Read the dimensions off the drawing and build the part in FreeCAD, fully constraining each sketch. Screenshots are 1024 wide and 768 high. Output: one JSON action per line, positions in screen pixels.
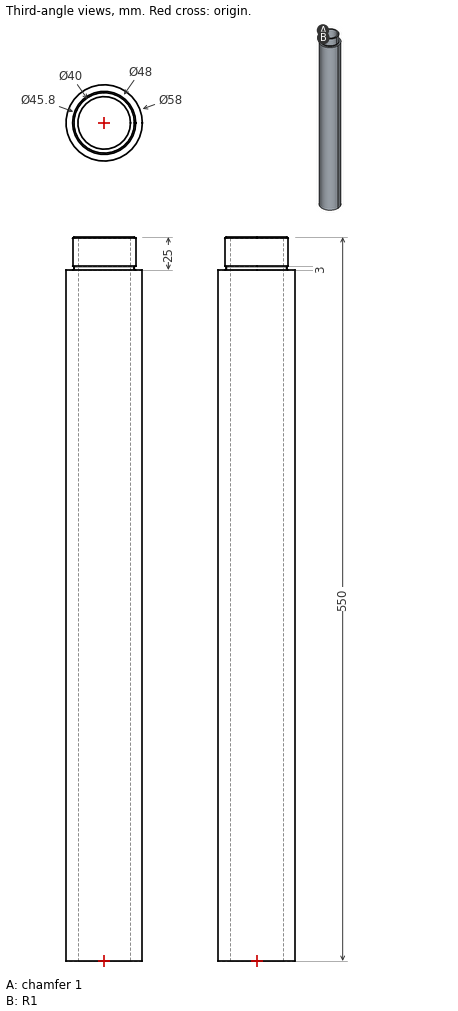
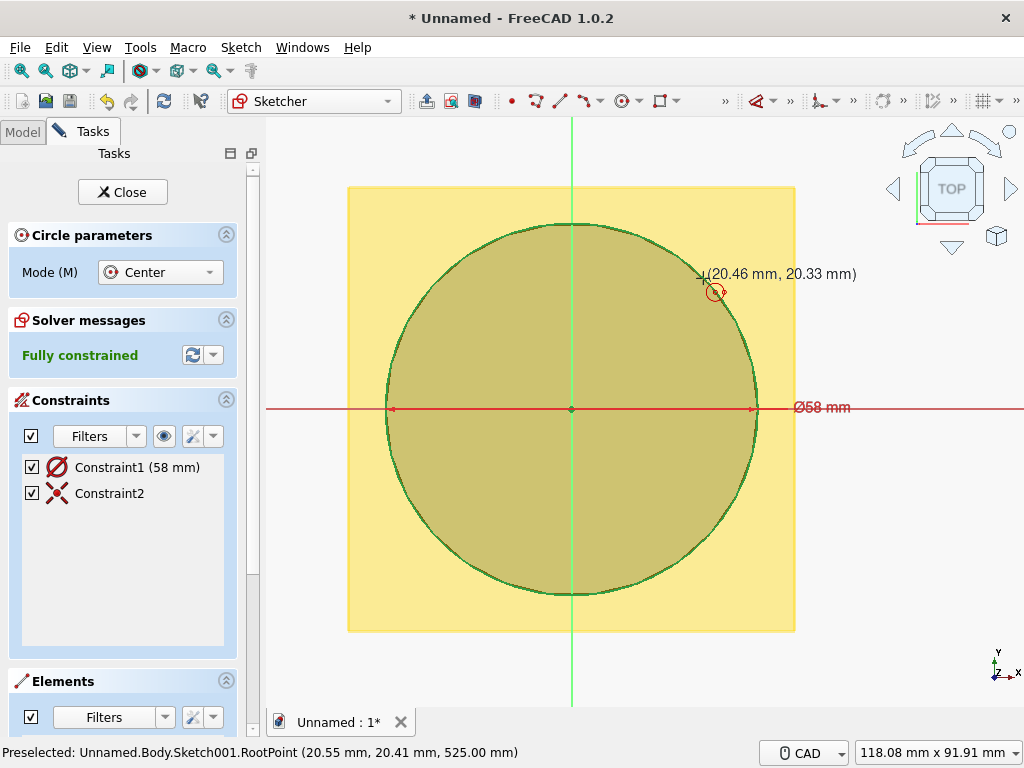
{"action": "left_click", "coordinate": [572, 409]}
{"action": "mouse_move", "coordinate": [681, 301]}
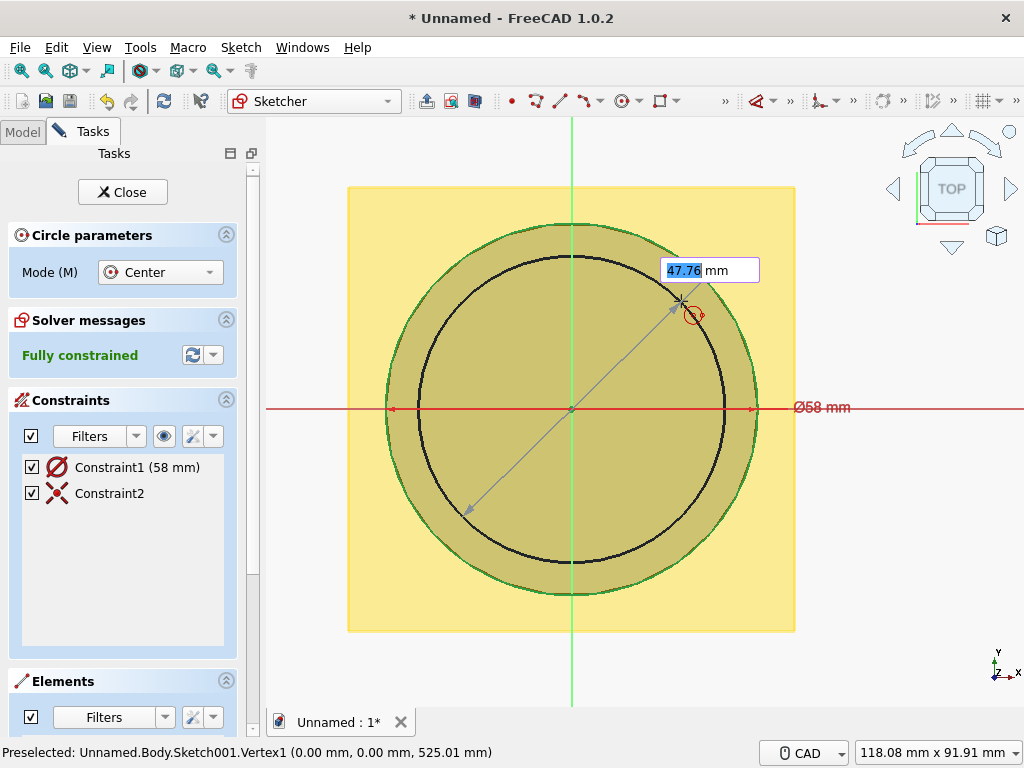
{"action": "type", "text": "48"}
{"action": "key", "text": "Return"}
{"action": "key", "text": "Escape"}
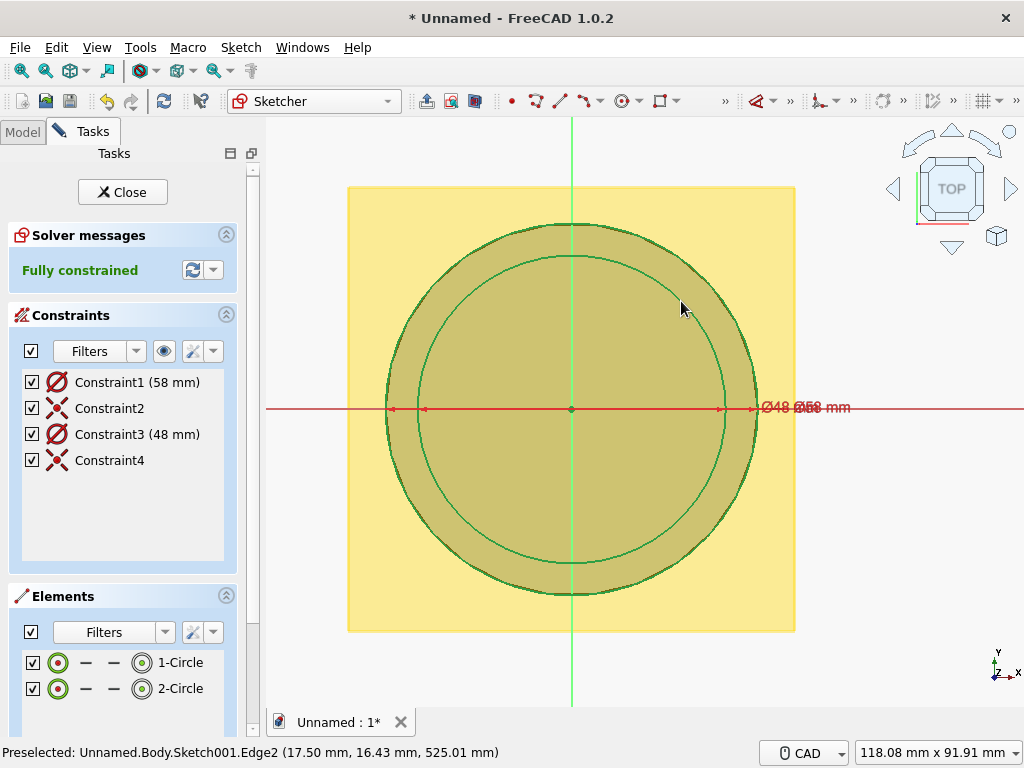
{"action": "left_click", "coordinate": [123, 192]}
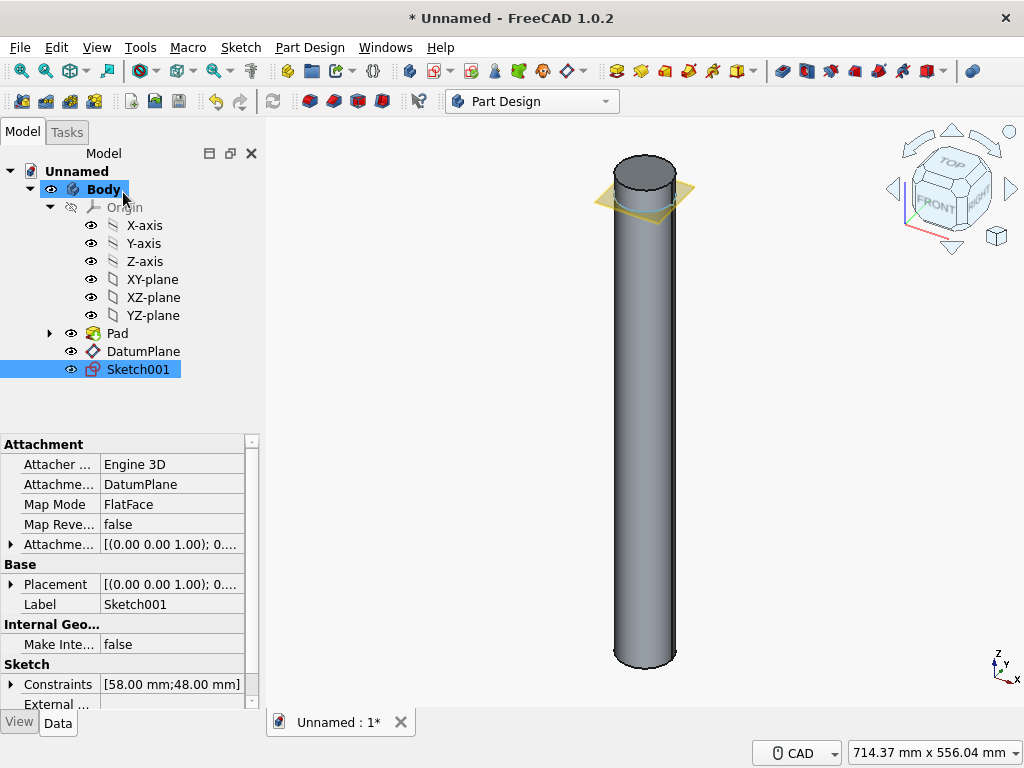
{"action": "left_click", "coordinate": [784, 72]}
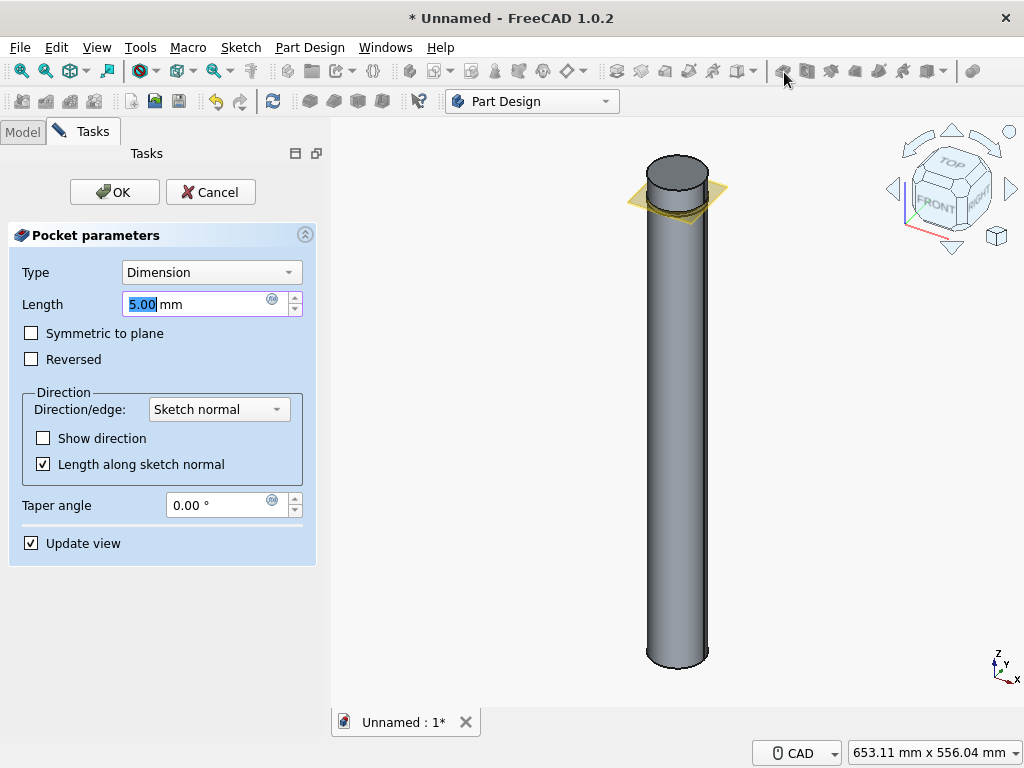
{"action": "type", "text": "25"}
{"action": "key", "text": "Tab"}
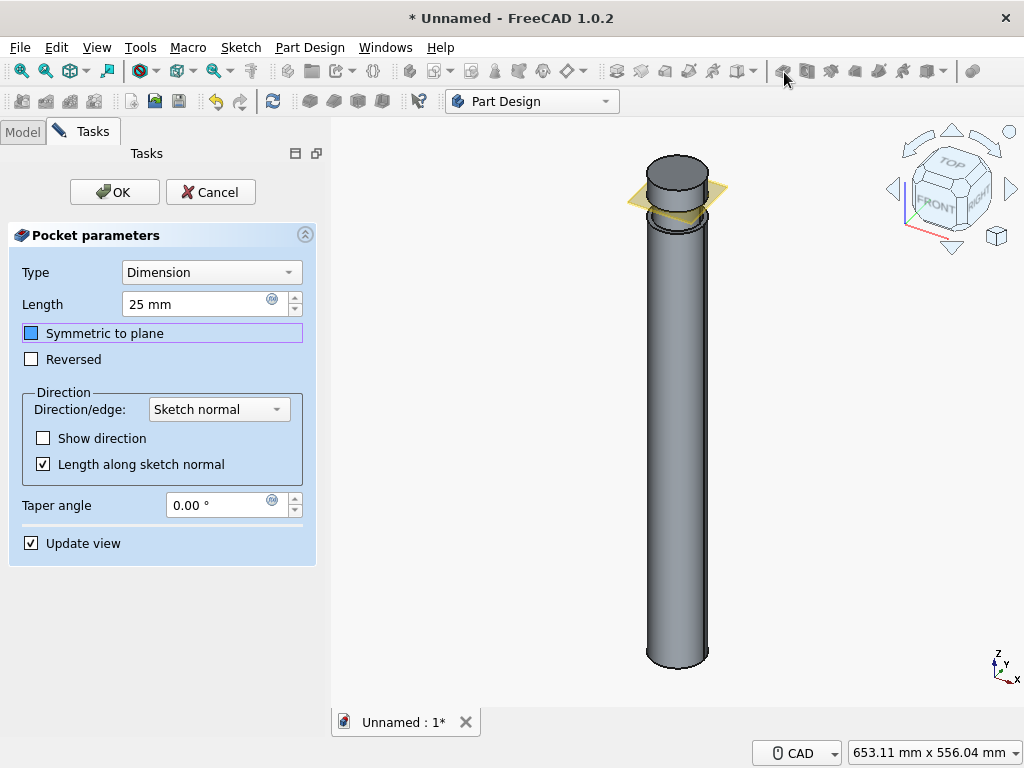
{"action": "left_click", "coordinate": [30, 359]}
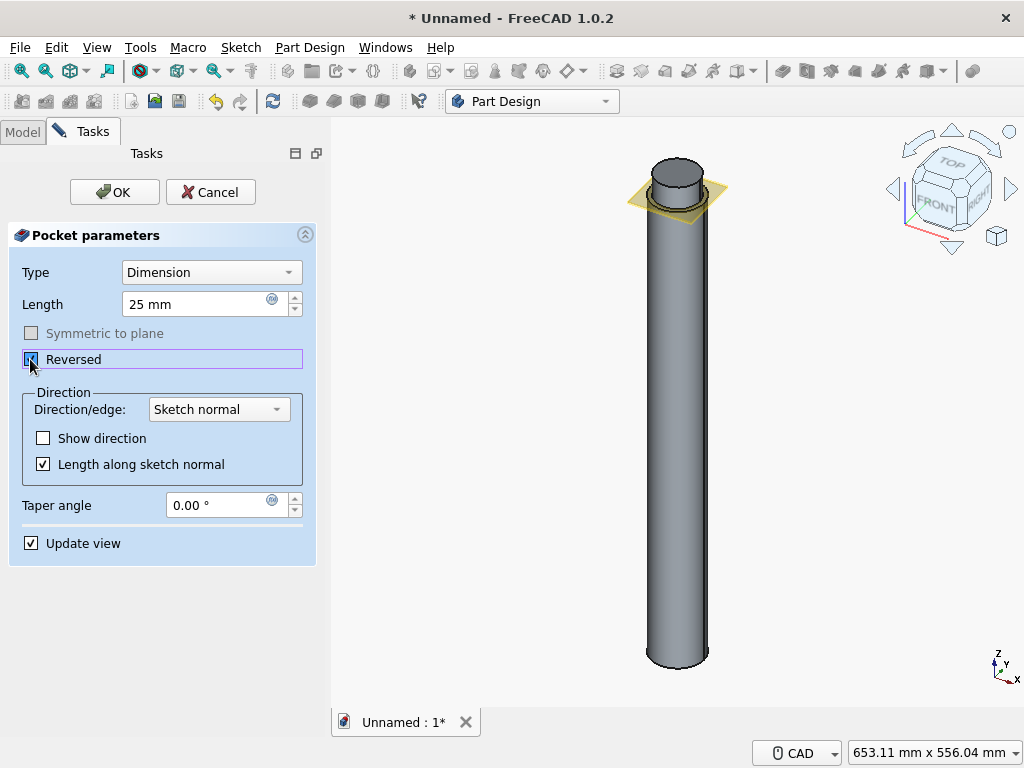
{"action": "left_click", "coordinate": [115, 192]}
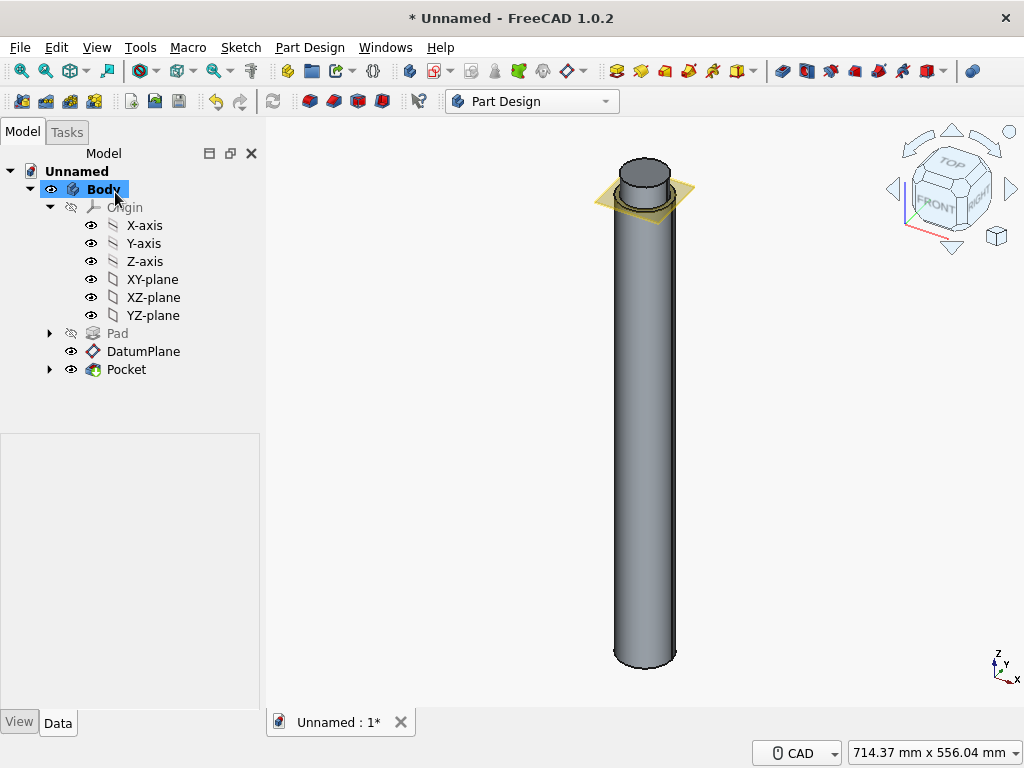
{"action": "left_click", "coordinate": [116, 351]}
{"action": "key", "text": "space"}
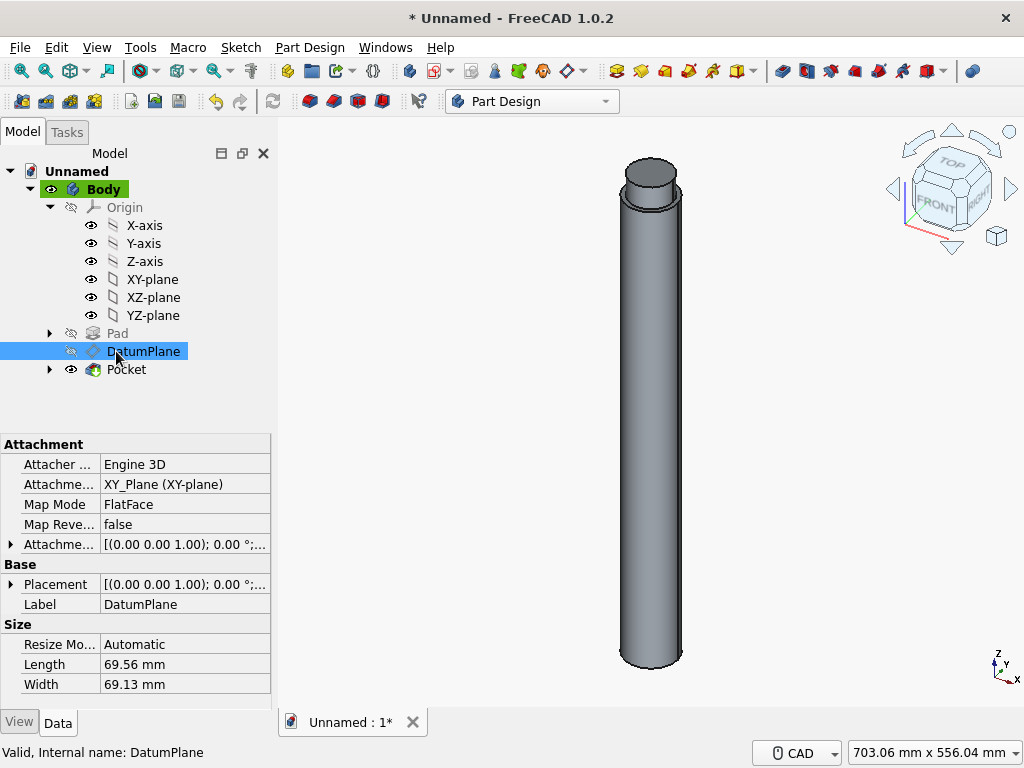
{"action": "left_click", "coordinate": [651, 172]}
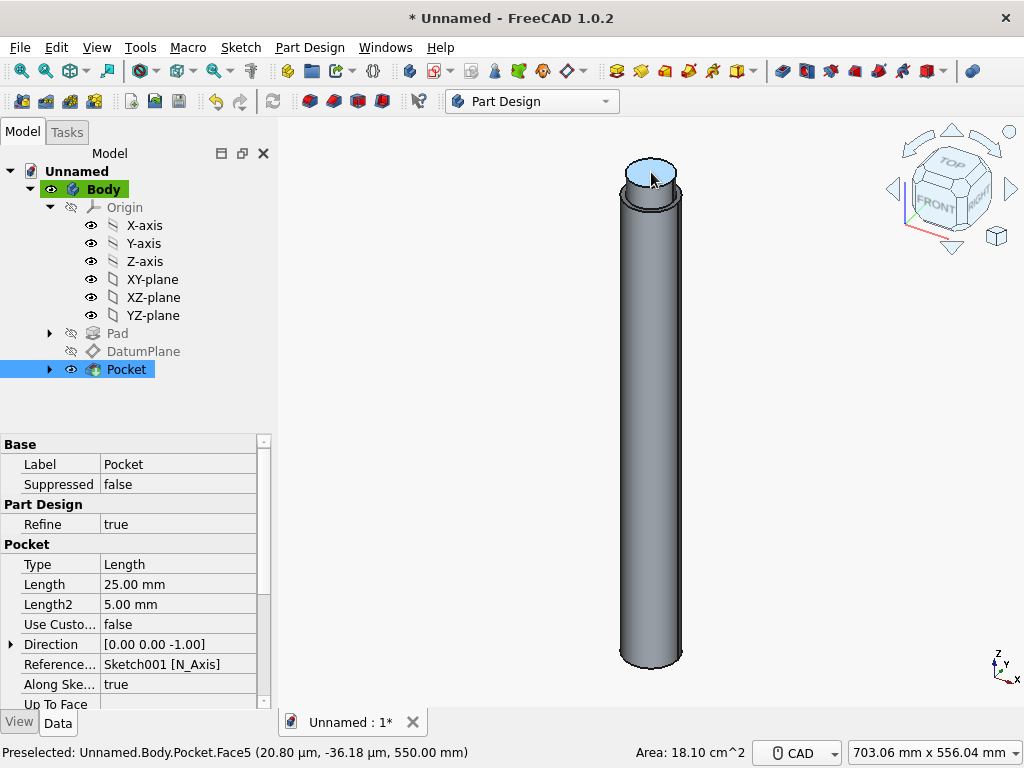
{"action": "left_click", "coordinate": [434, 72]}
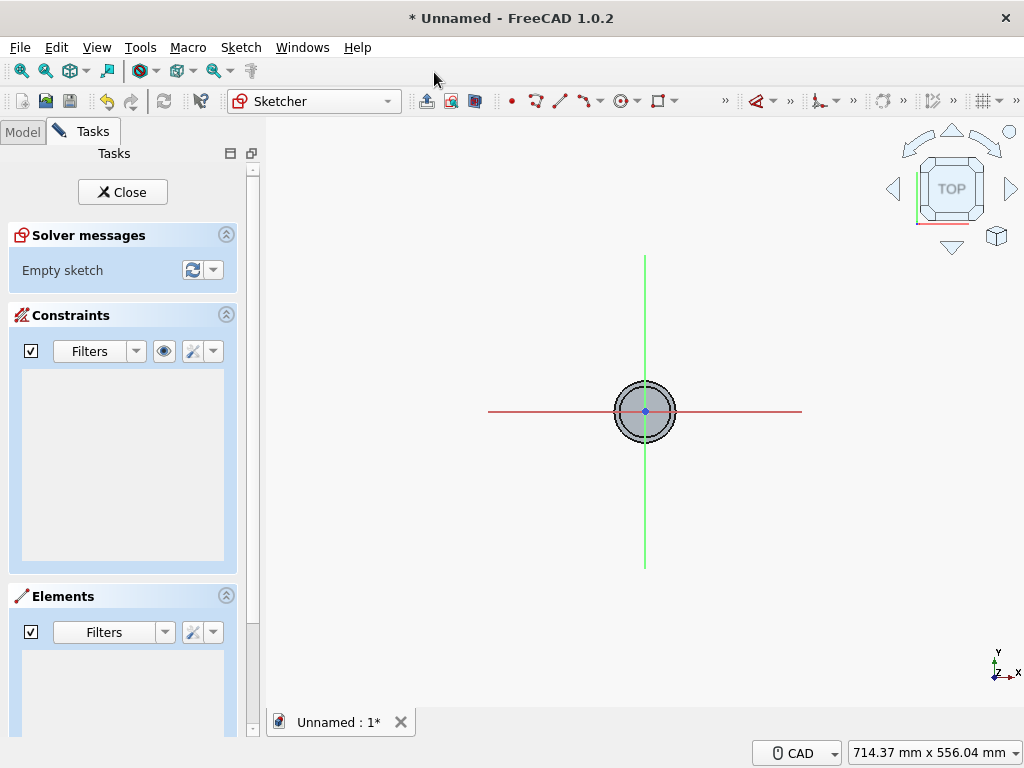
{"action": "scroll", "coordinate": [654, 412], "scroll_direction": "up", "scroll_amount": 11}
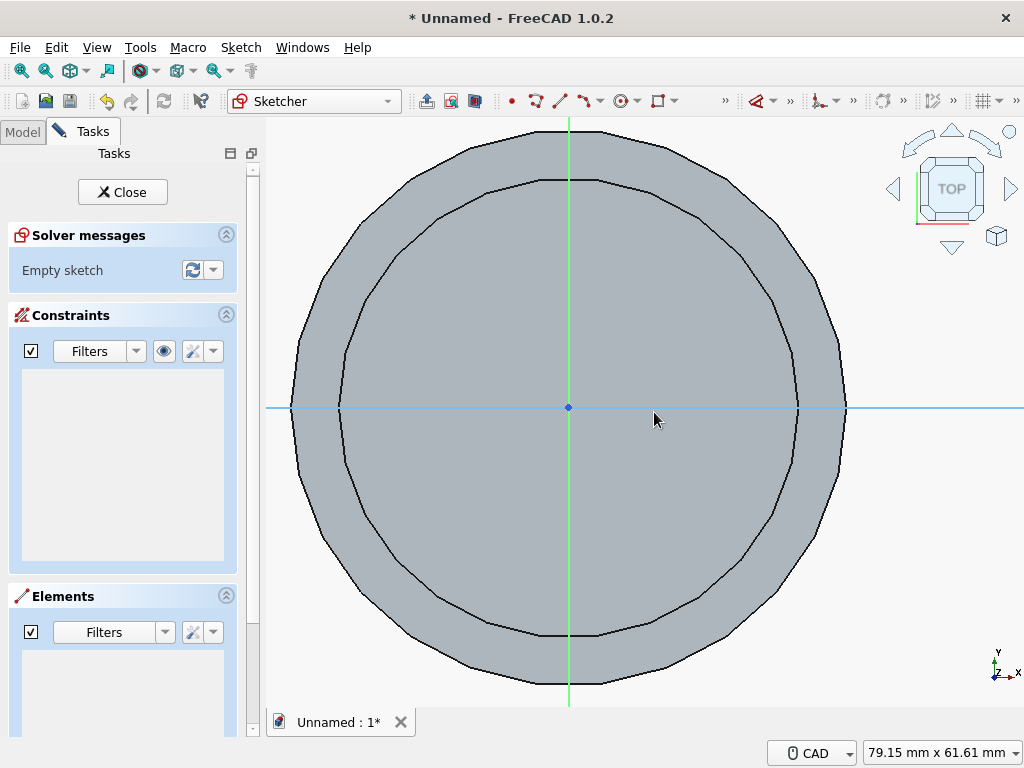
{"action": "left_click", "coordinate": [622, 102]}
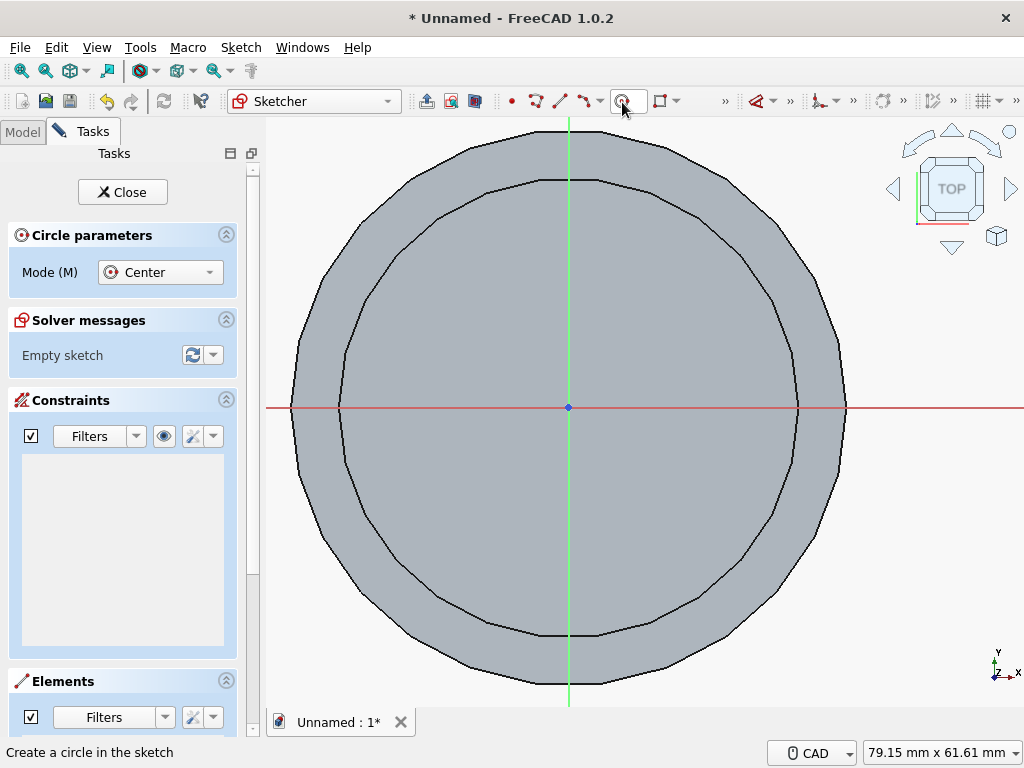
{"action": "left_click", "coordinate": [569, 408]}
{"action": "mouse_move", "coordinate": [704, 273]}